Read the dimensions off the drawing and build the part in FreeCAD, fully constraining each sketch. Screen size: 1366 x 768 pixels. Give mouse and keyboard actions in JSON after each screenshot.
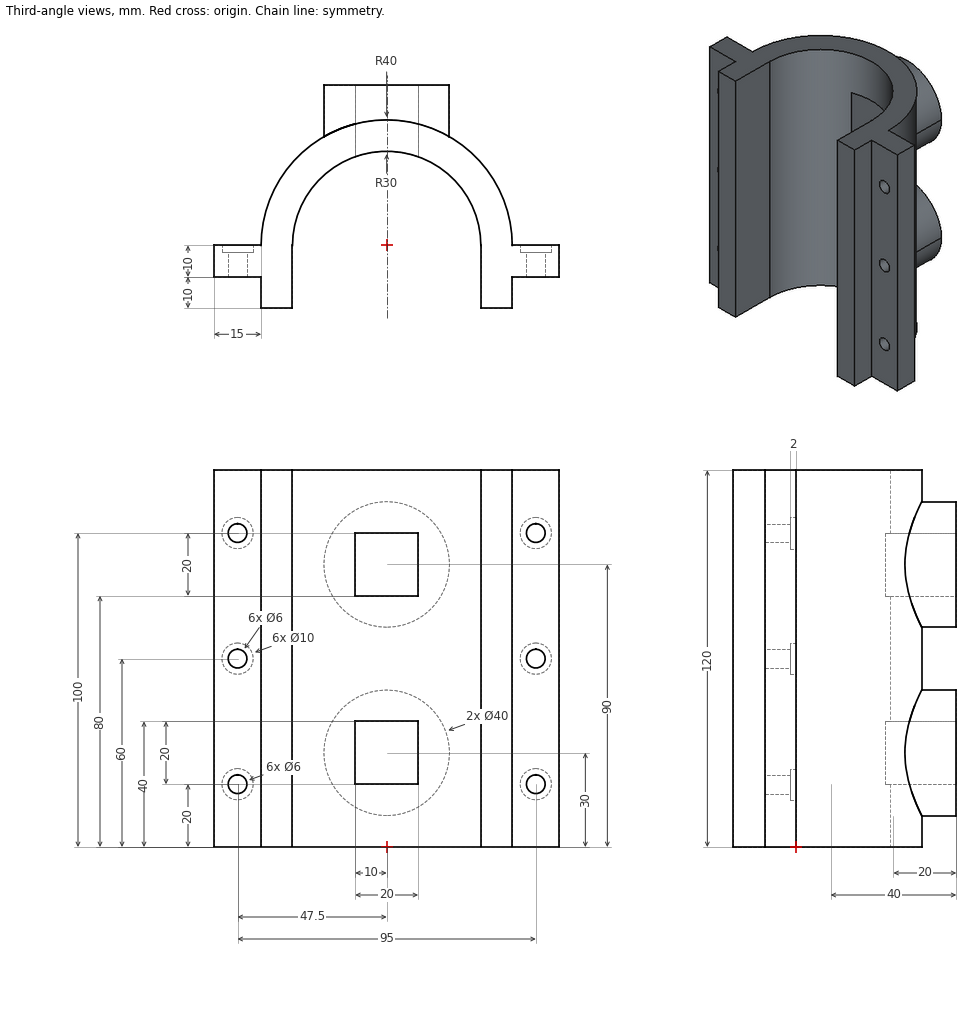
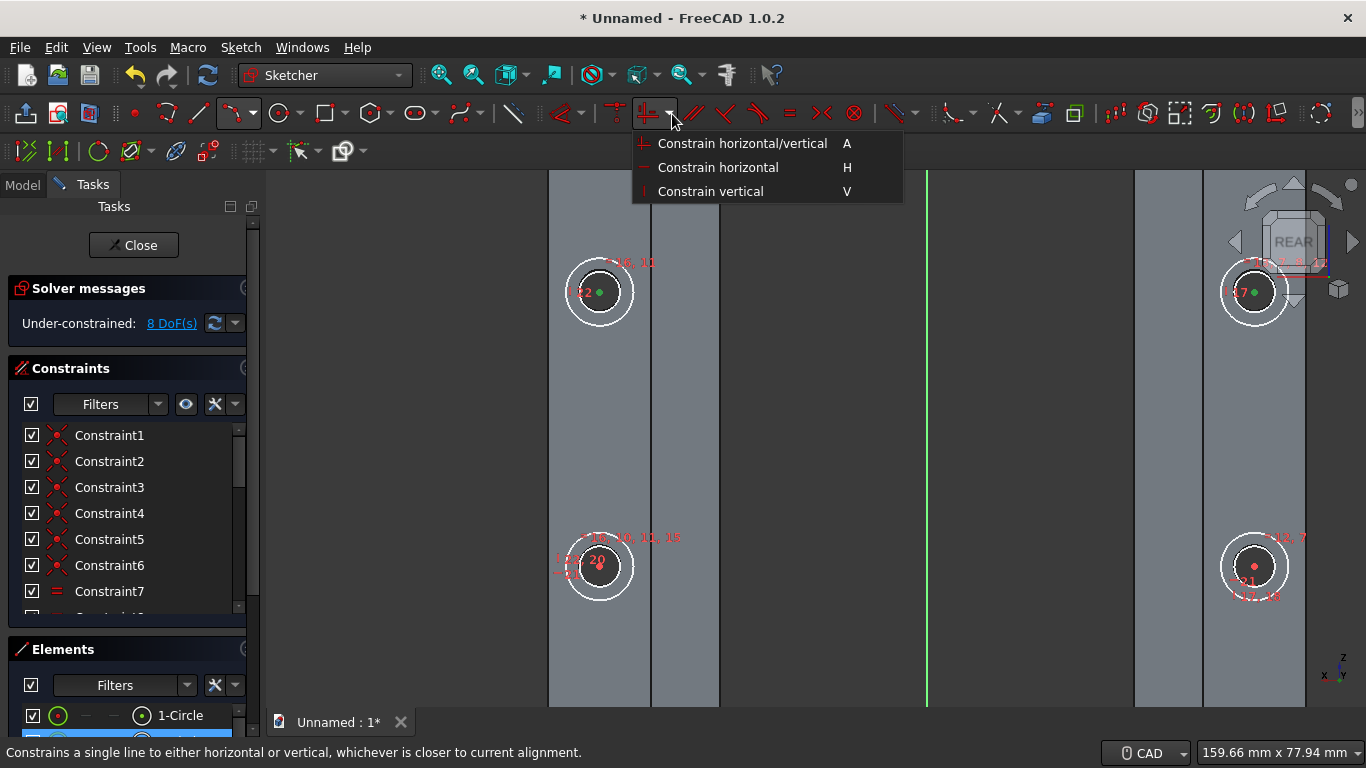
{"action": "left_click", "coordinate": [768, 167]}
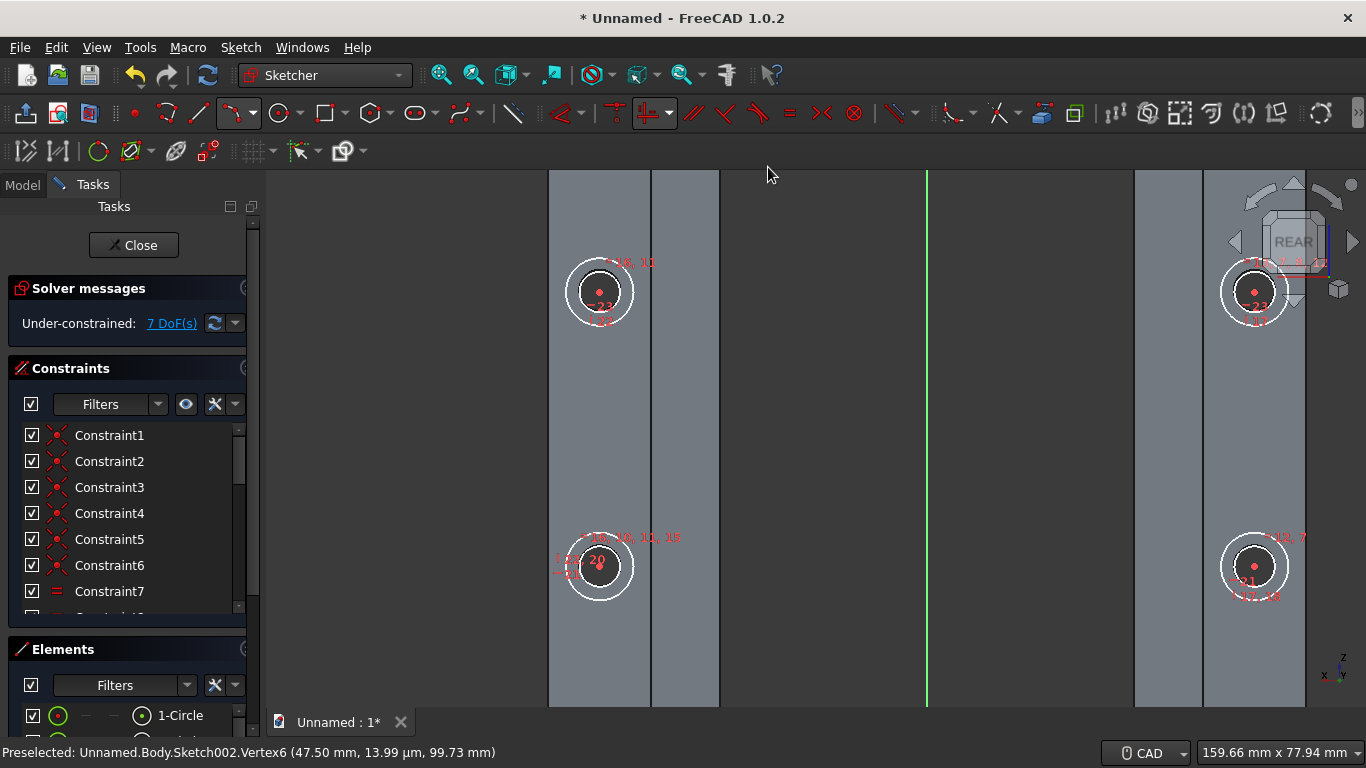
{"action": "left_click", "coordinate": [560, 114]}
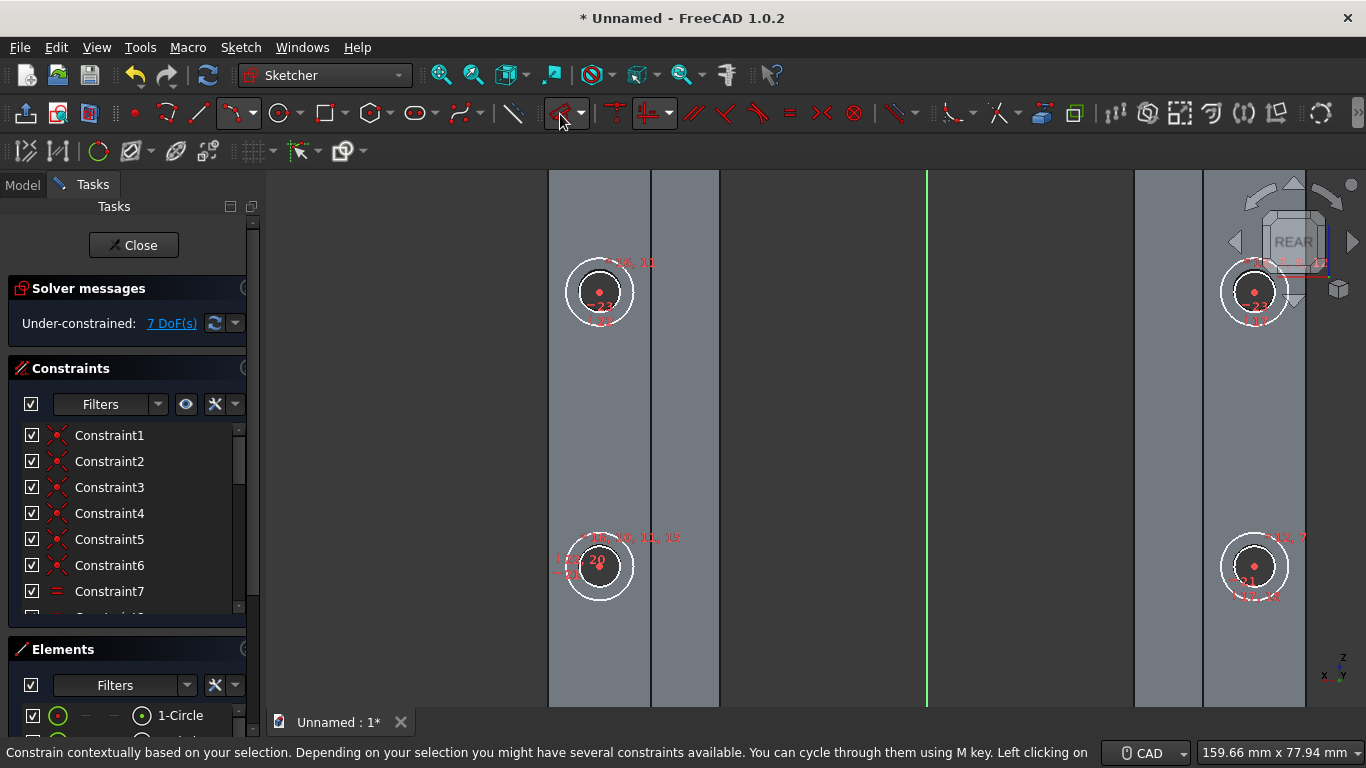
{"action": "scroll", "coordinate": [601, 292], "scroll_direction": "down", "scroll_amount": 4}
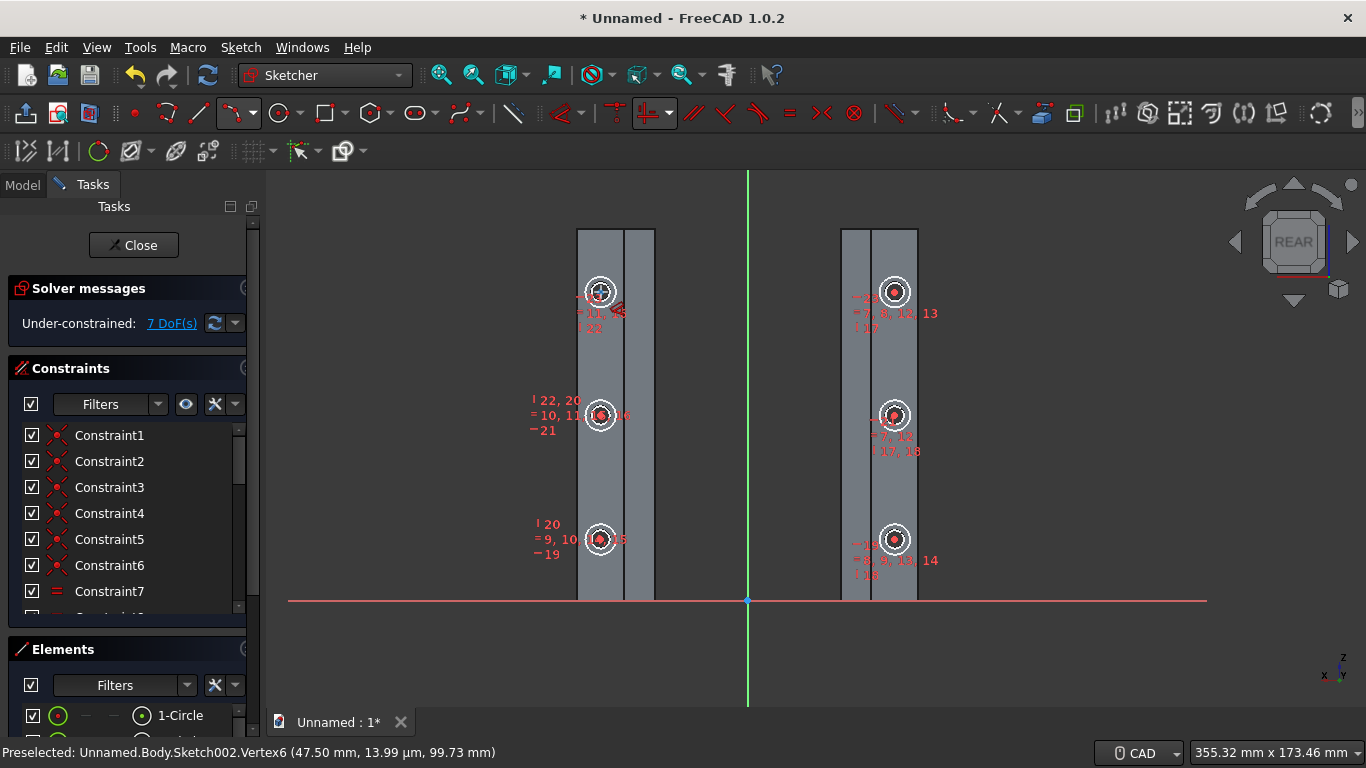
{"action": "scroll", "coordinate": [906, 405], "scroll_direction": "up", "scroll_amount": 5}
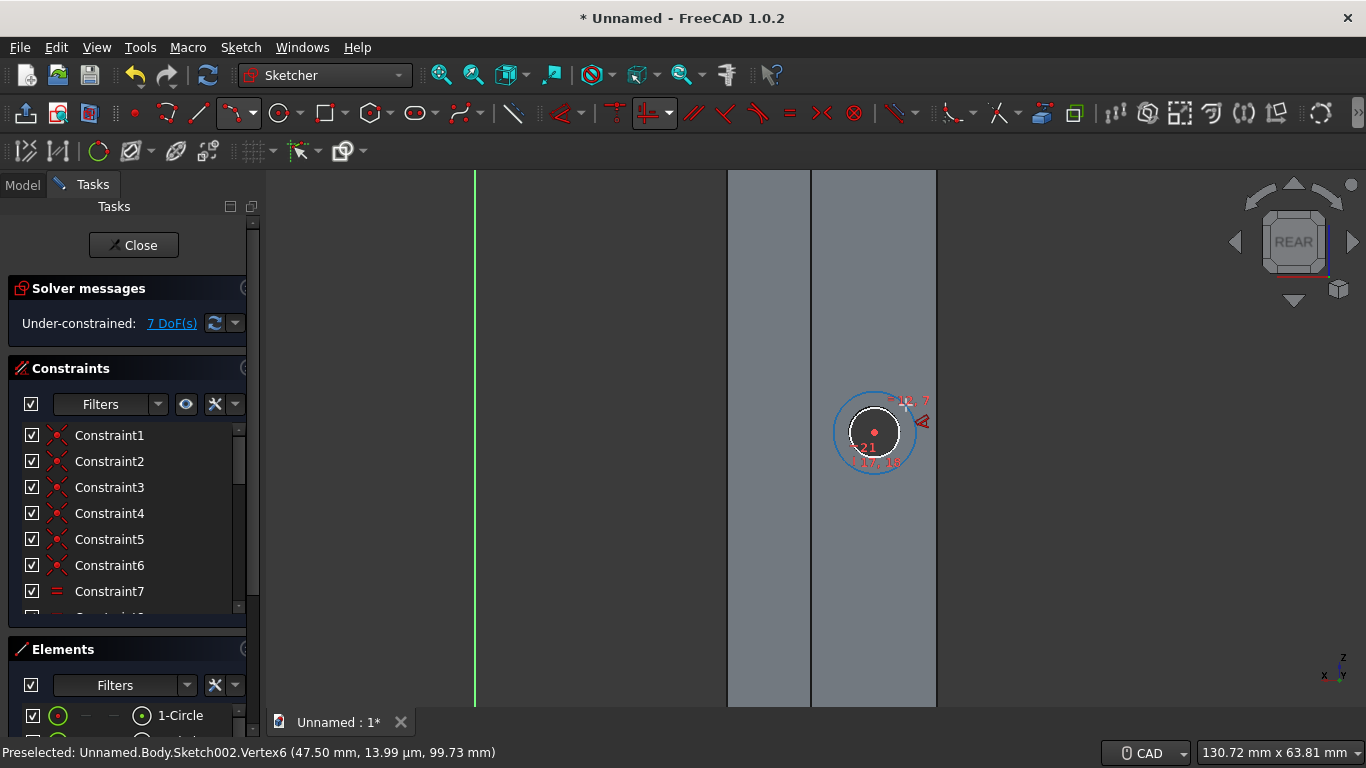
{"action": "left_click", "coordinate": [904, 404]}
{"action": "left_click", "coordinate": [927, 382]}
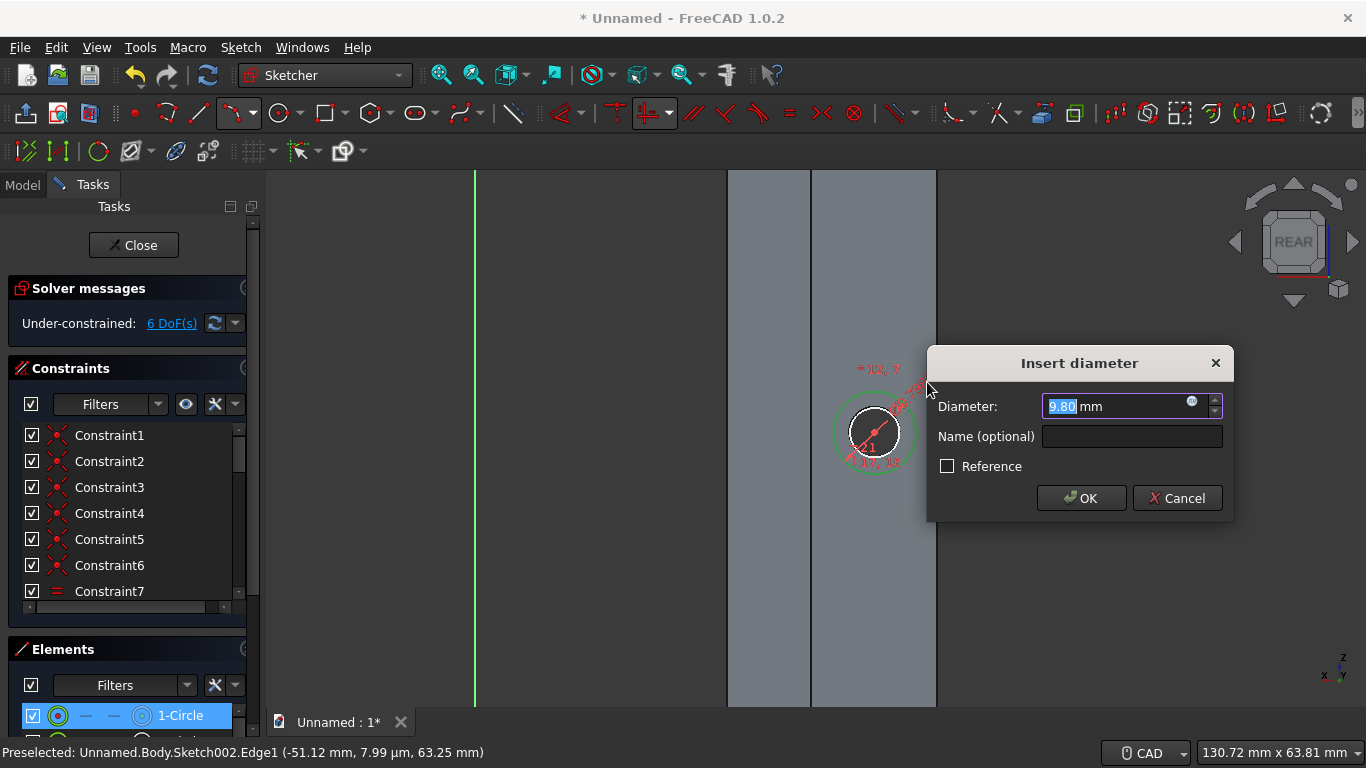
{"action": "type", "text": "10"}
{"action": "key", "text": "Return"}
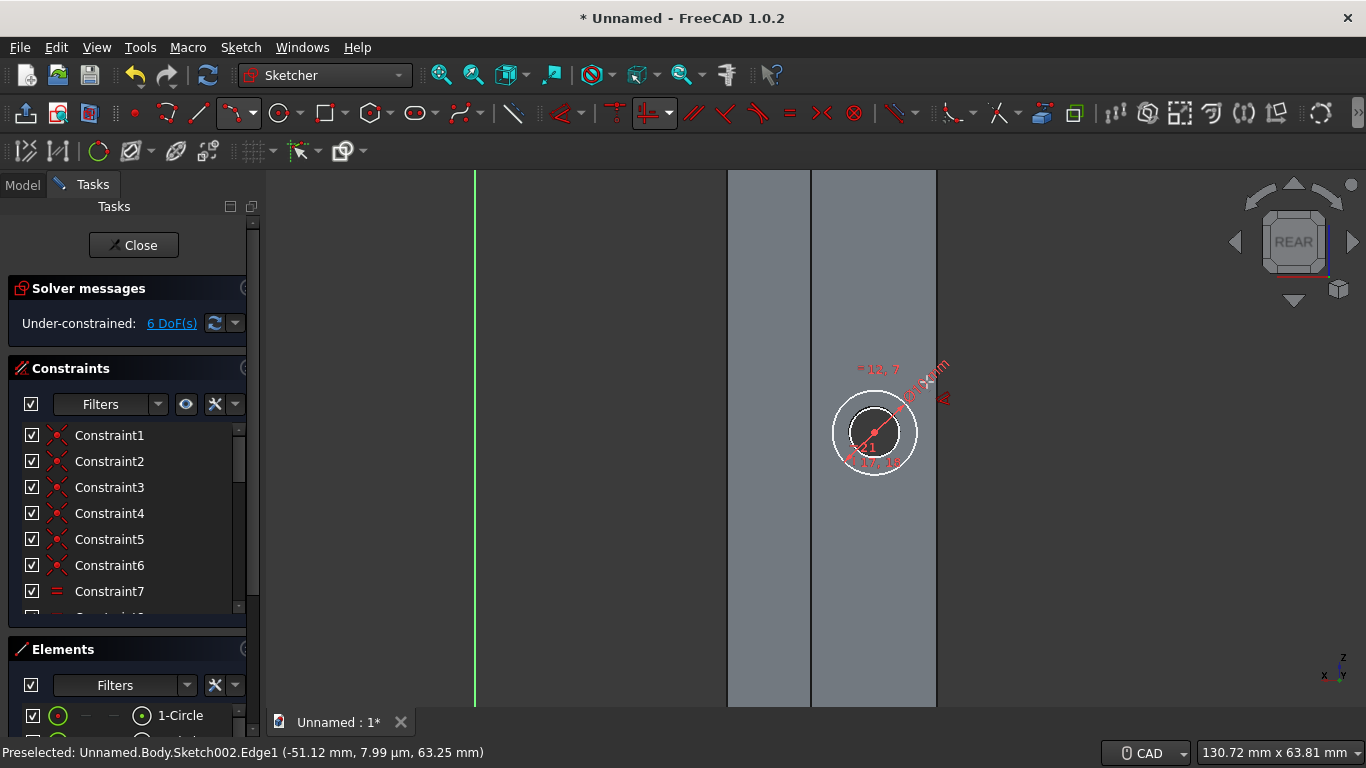
{"action": "left_click", "coordinate": [892, 415]}
{"action": "left_click", "coordinate": [929, 416]}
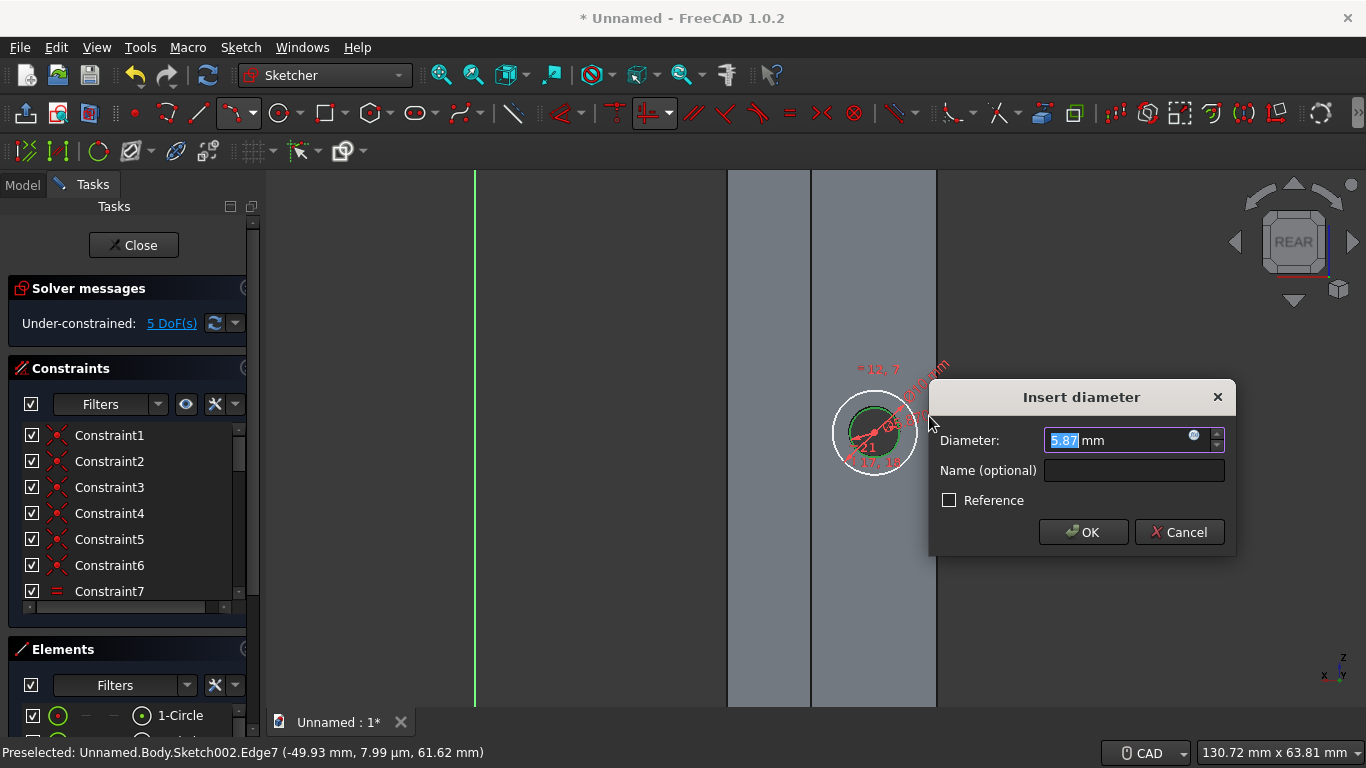
{"action": "type", "text": "6"}
{"action": "key", "text": "Return"}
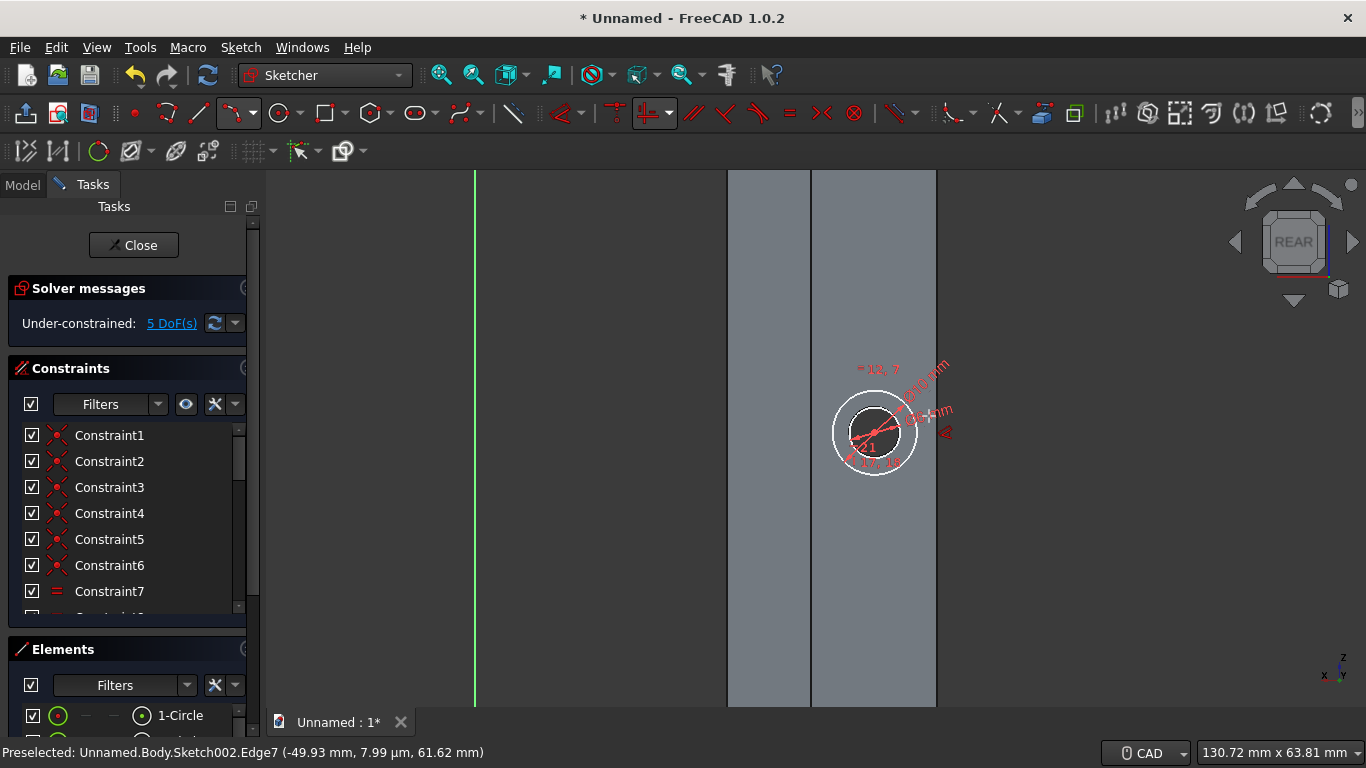
{"action": "left_click", "coordinate": [875, 433]}
{"action": "left_click", "coordinate": [909, 556]}